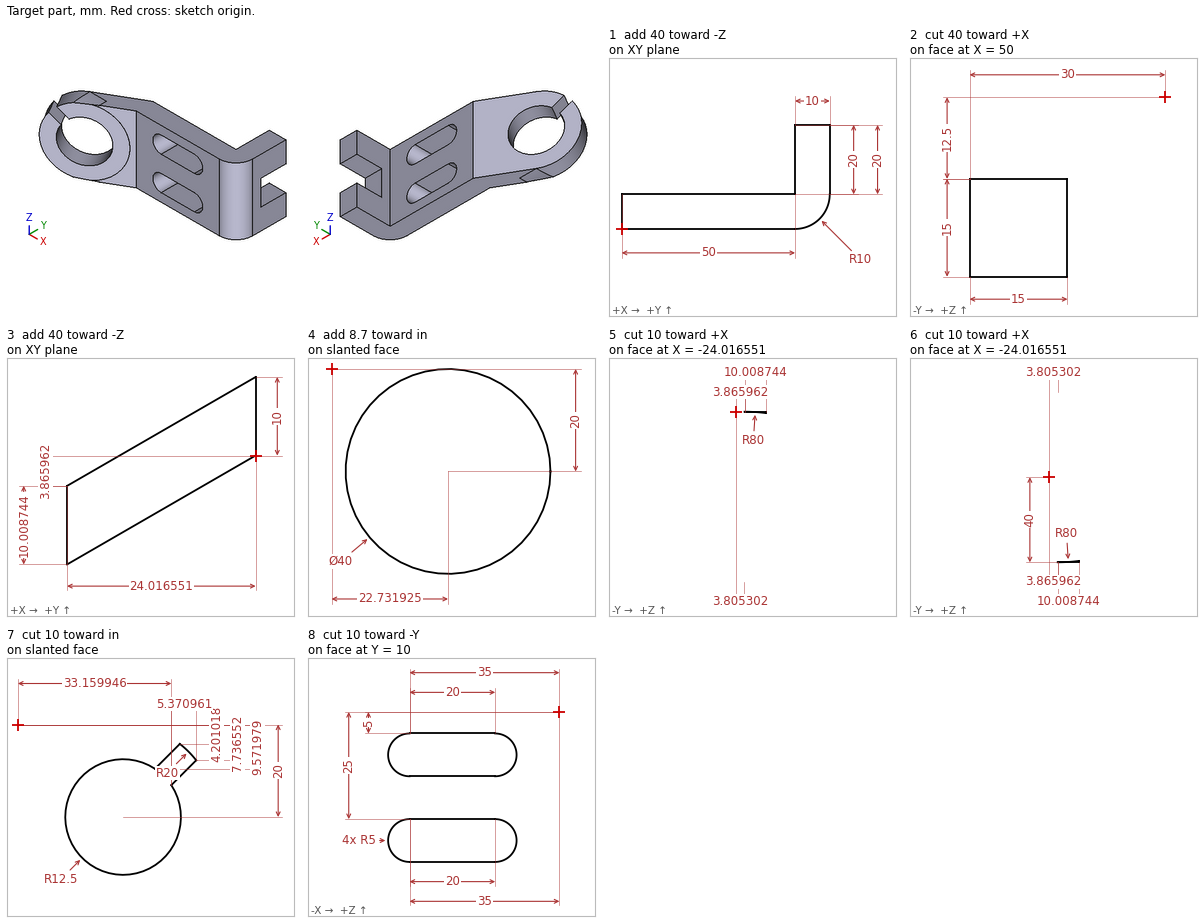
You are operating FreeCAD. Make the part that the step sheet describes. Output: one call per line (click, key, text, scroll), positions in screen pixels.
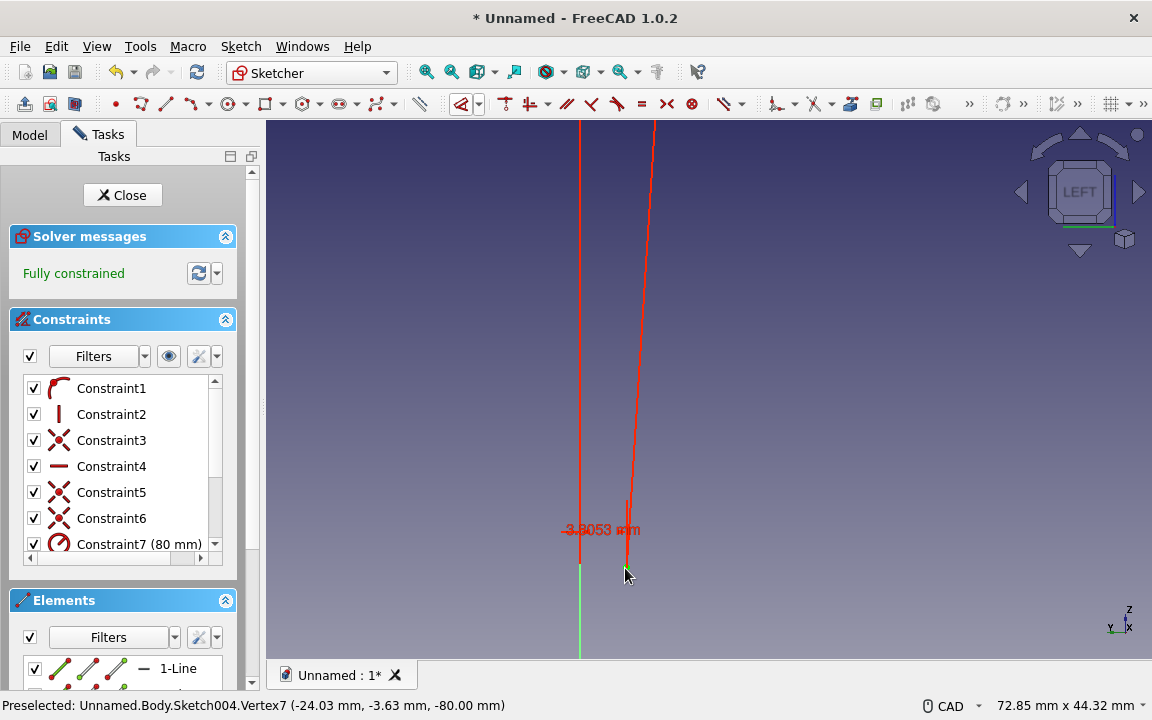
click(123, 195)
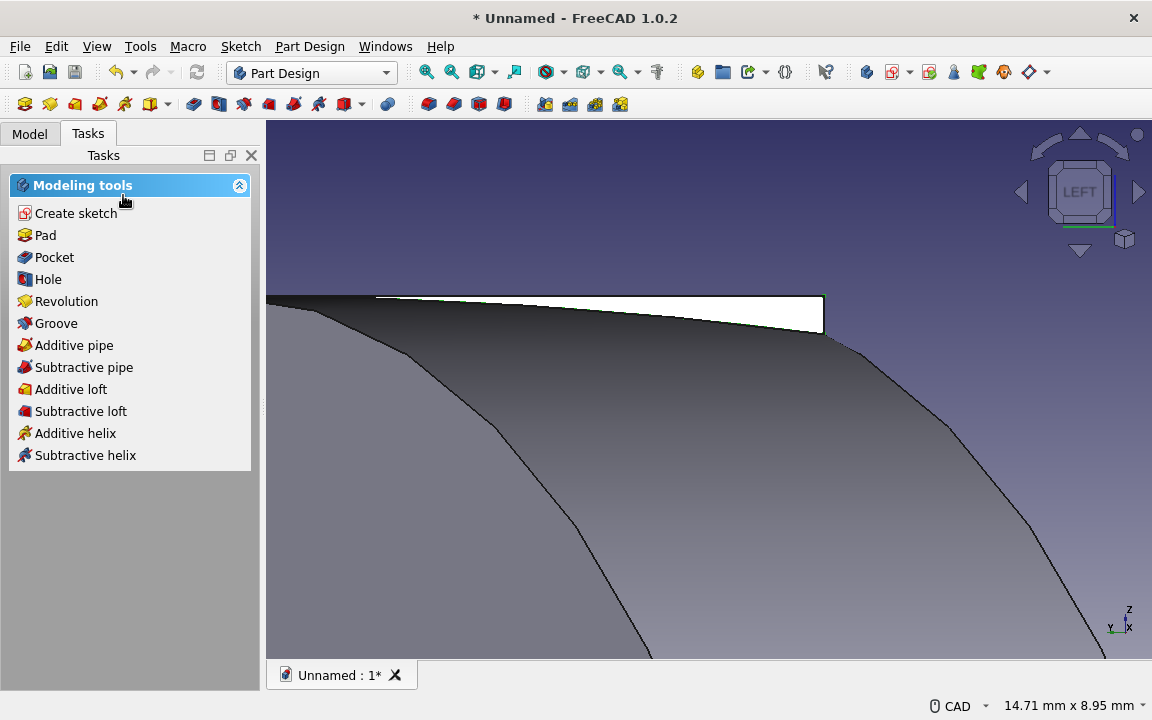
click(194, 104)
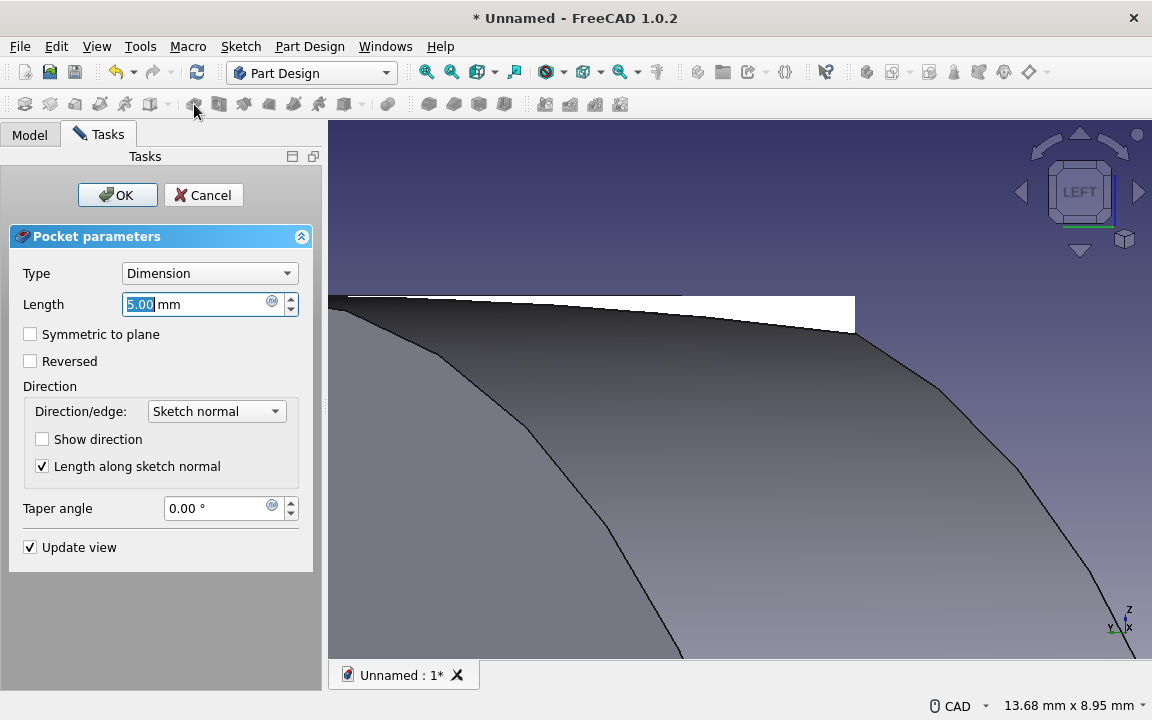
text(10)
key(Tab)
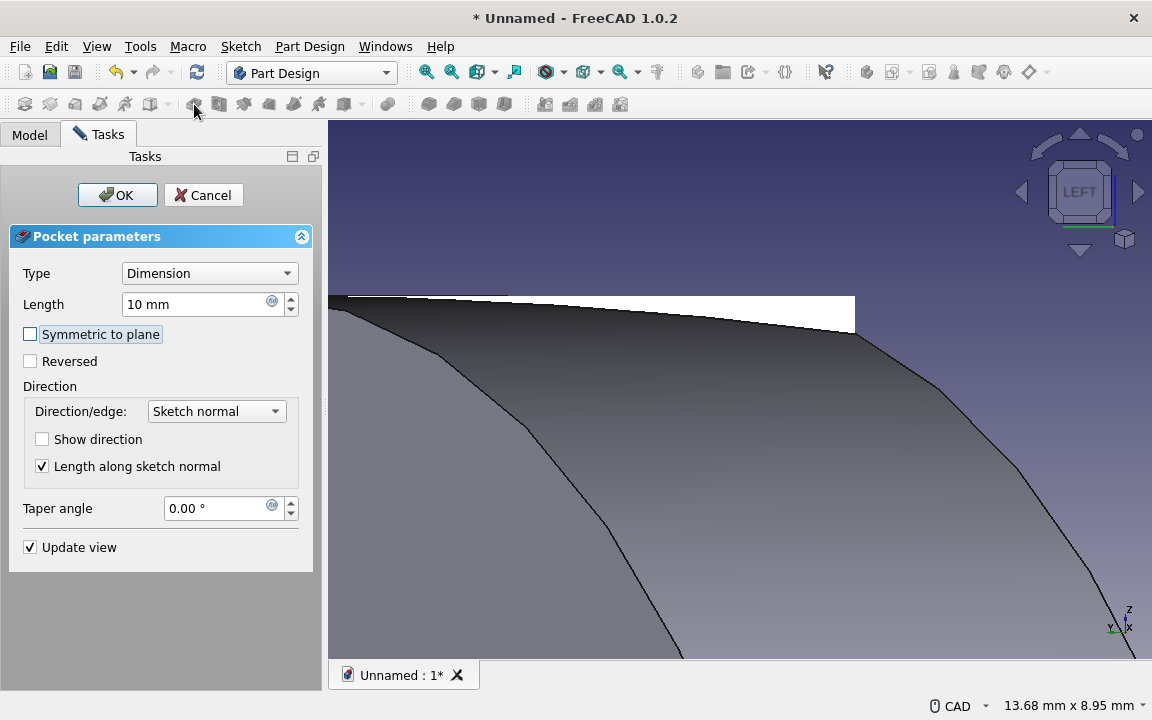
click(118, 195)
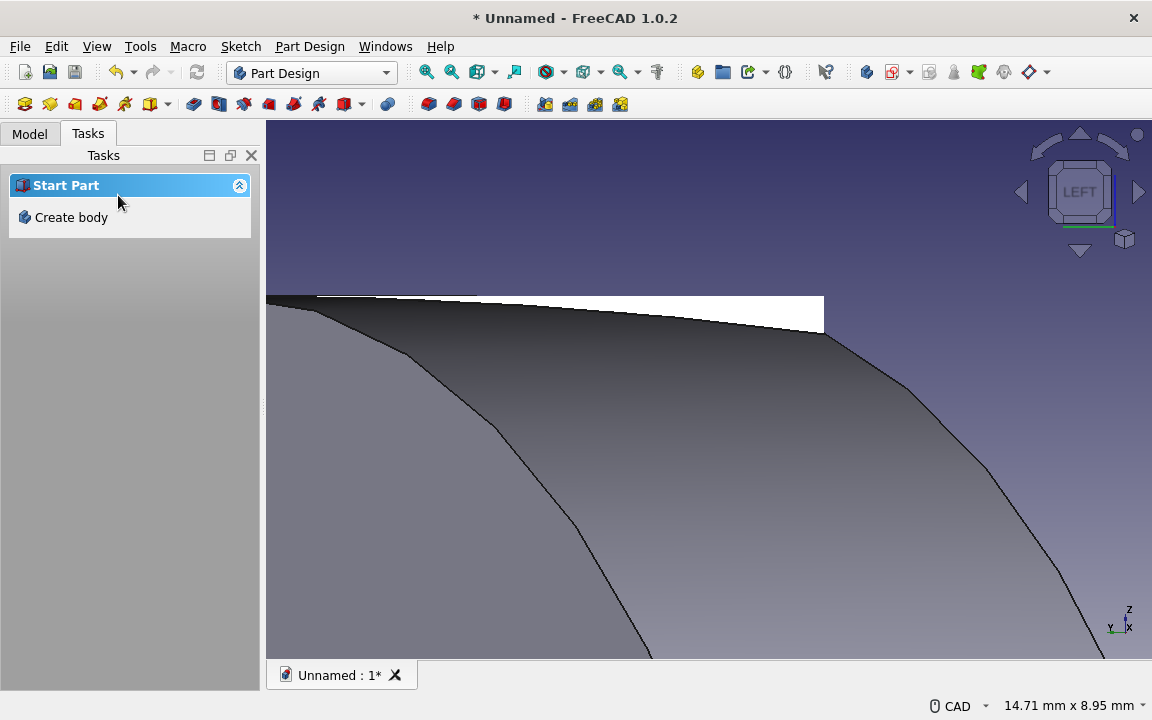
click(427, 72)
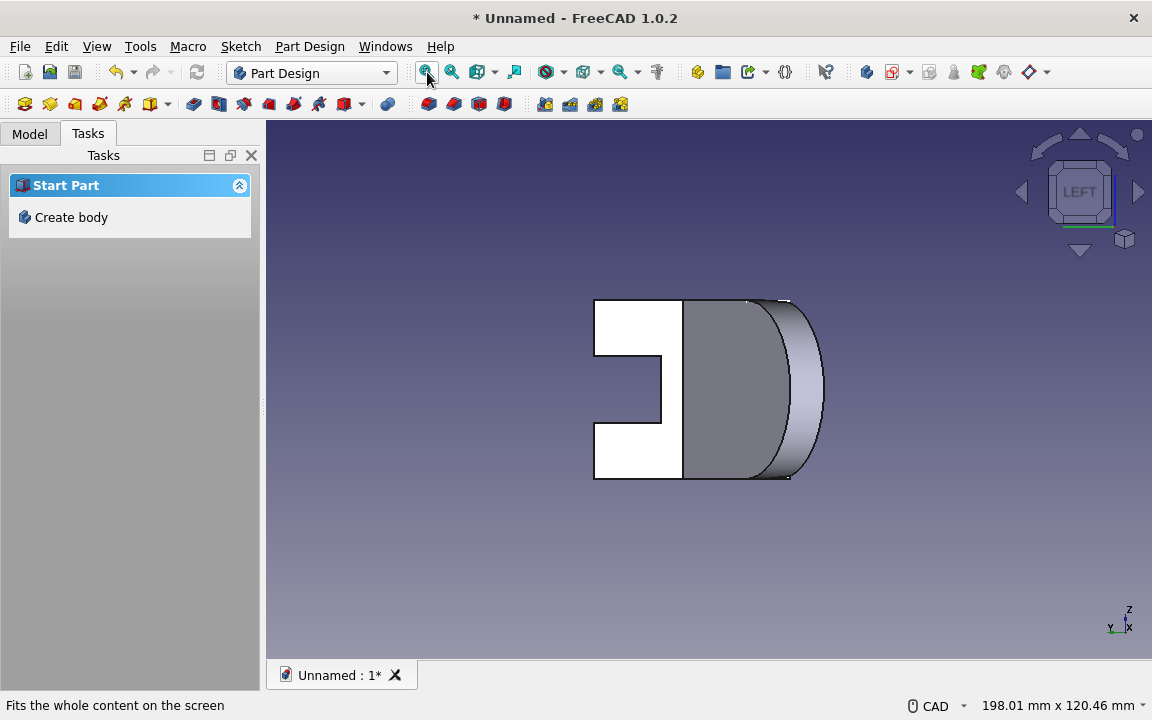
scroll(787, 477, up, 13)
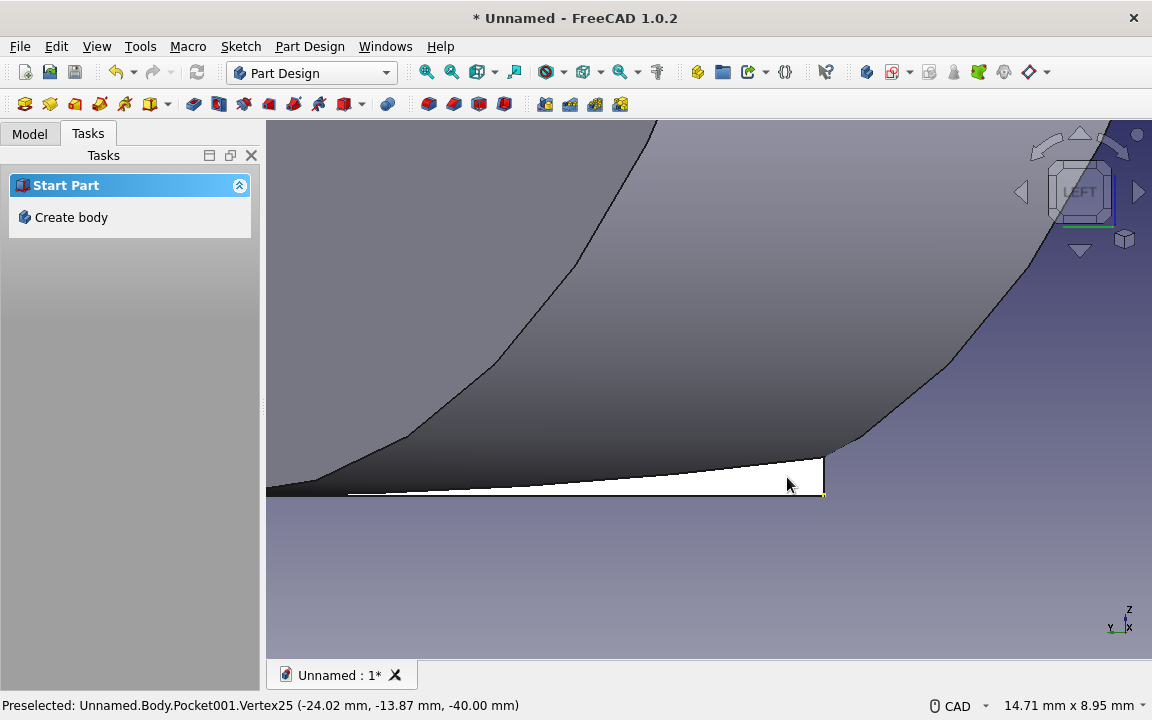
click(781, 475)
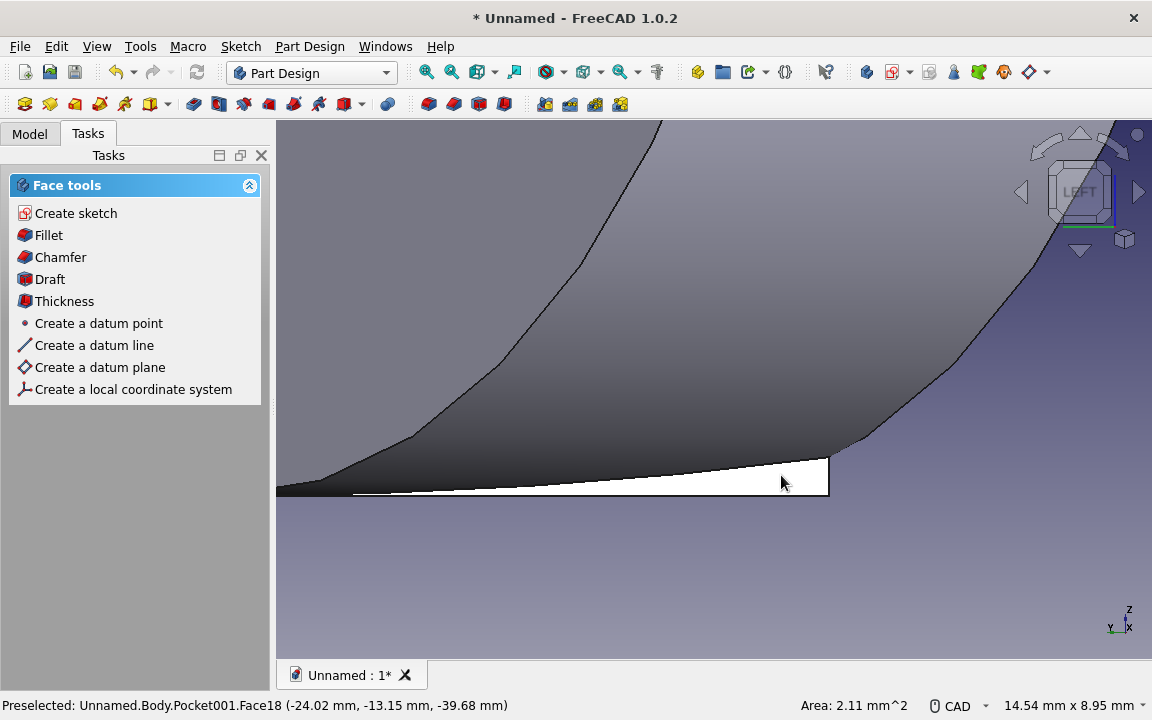
click(892, 72)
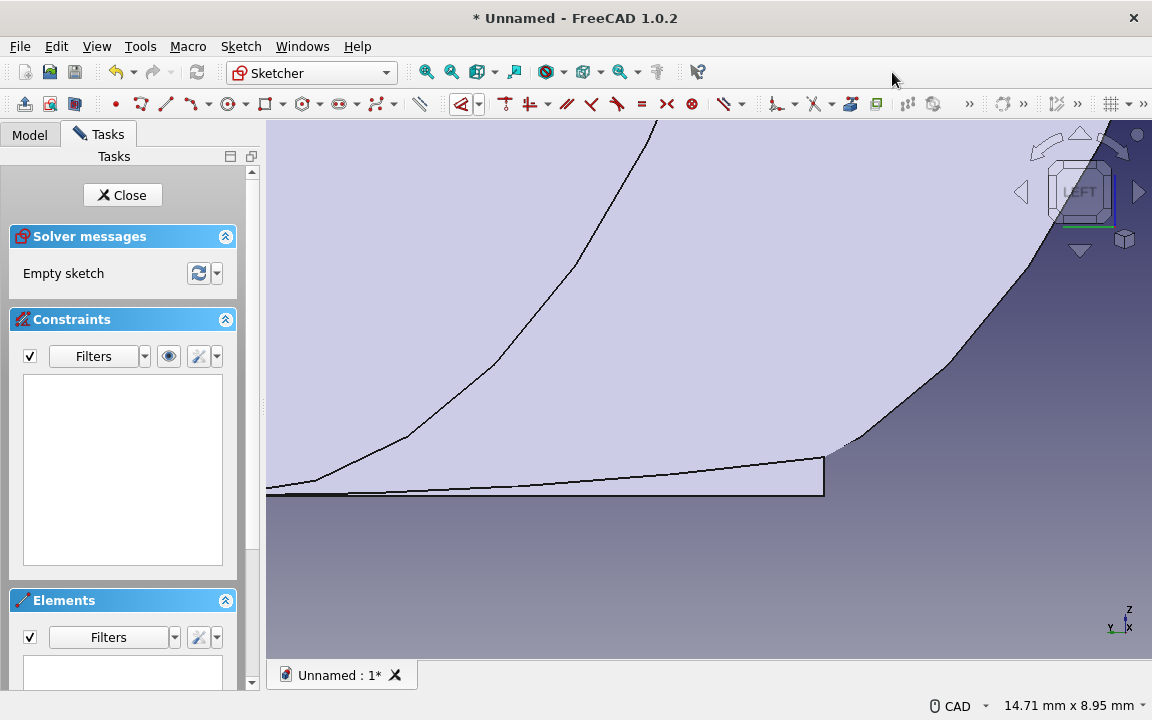
click(75, 104)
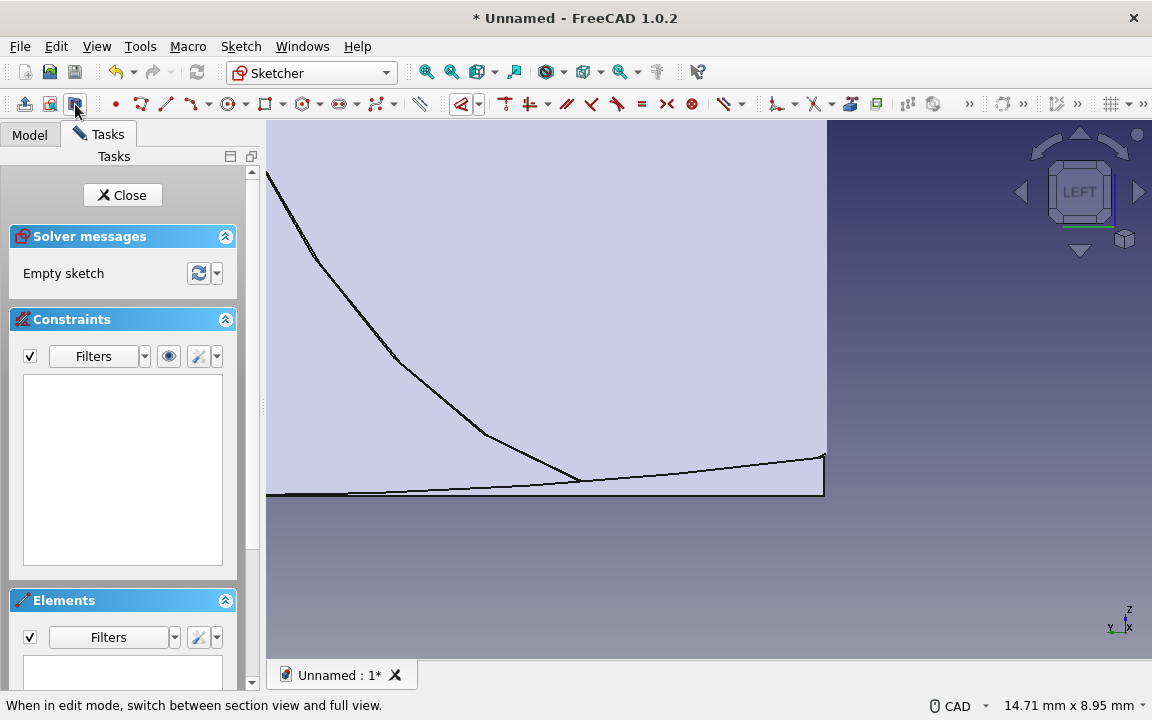
scroll(987, 148, down, 1)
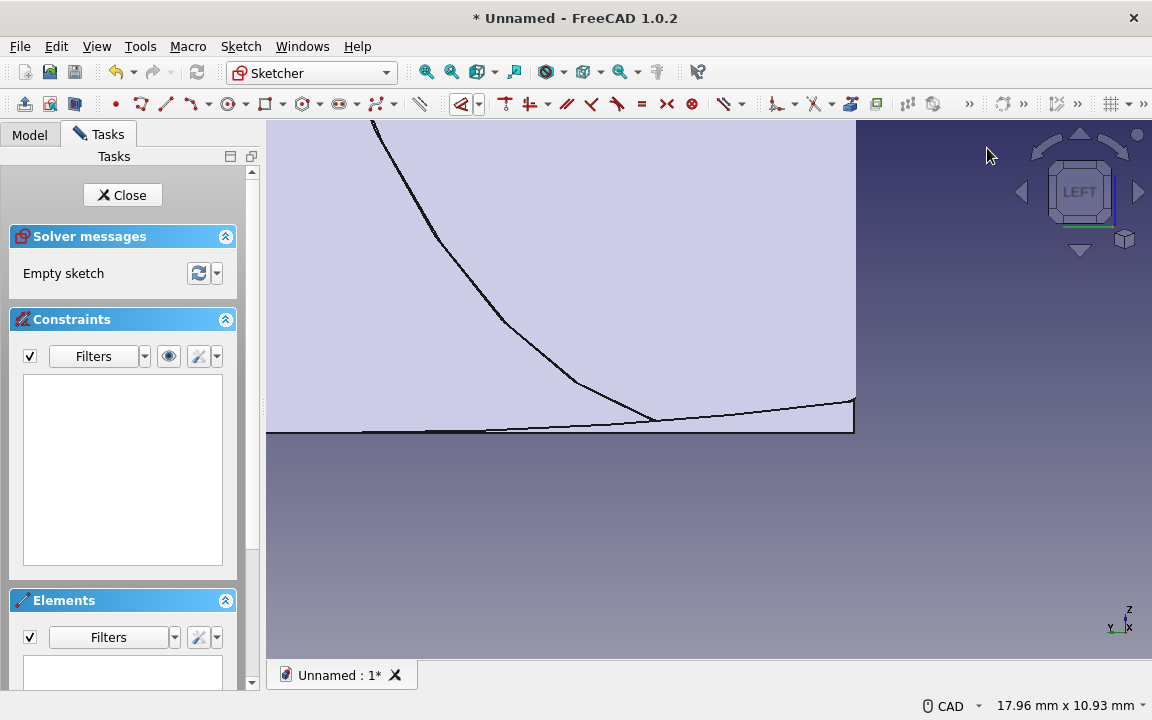
key(g)
key(m)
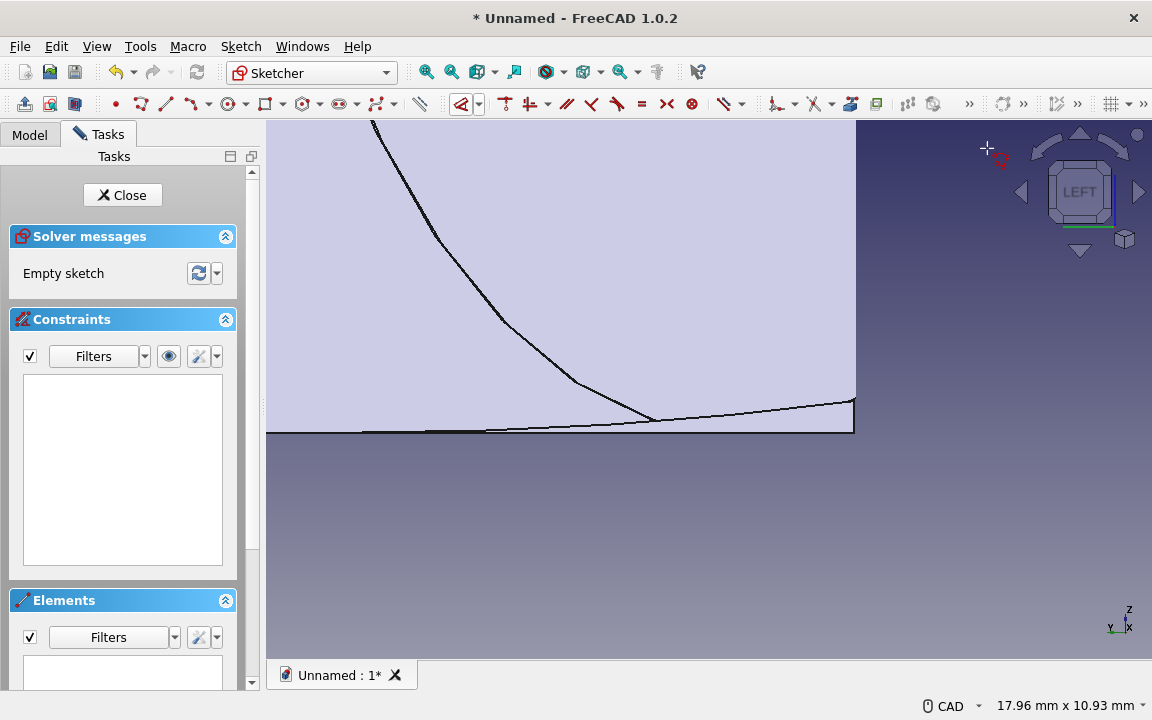
click(360, 433)
click(854, 433)
click(854, 401)
right_click(854, 401)